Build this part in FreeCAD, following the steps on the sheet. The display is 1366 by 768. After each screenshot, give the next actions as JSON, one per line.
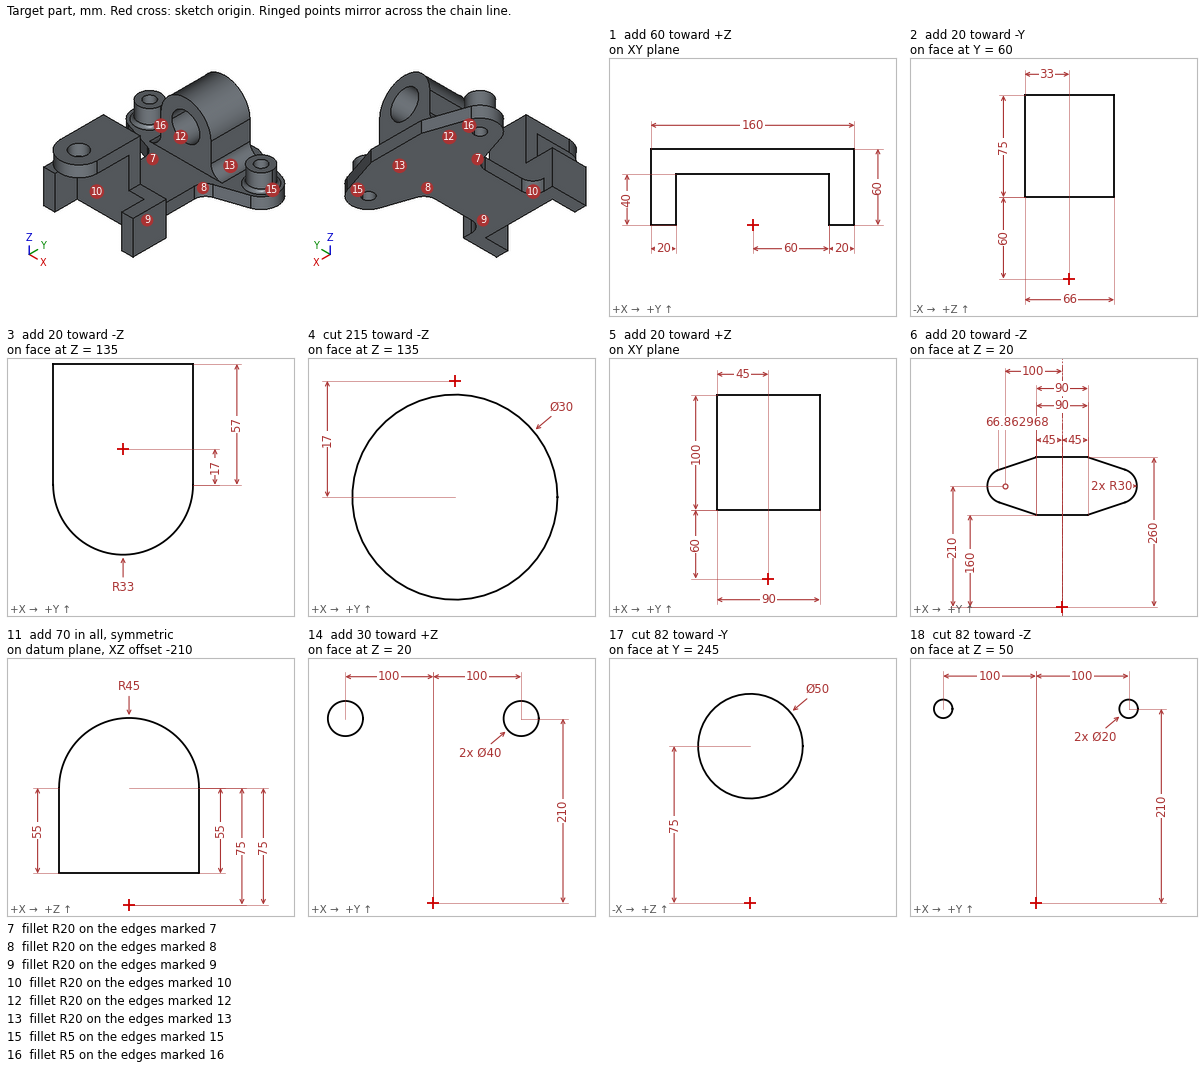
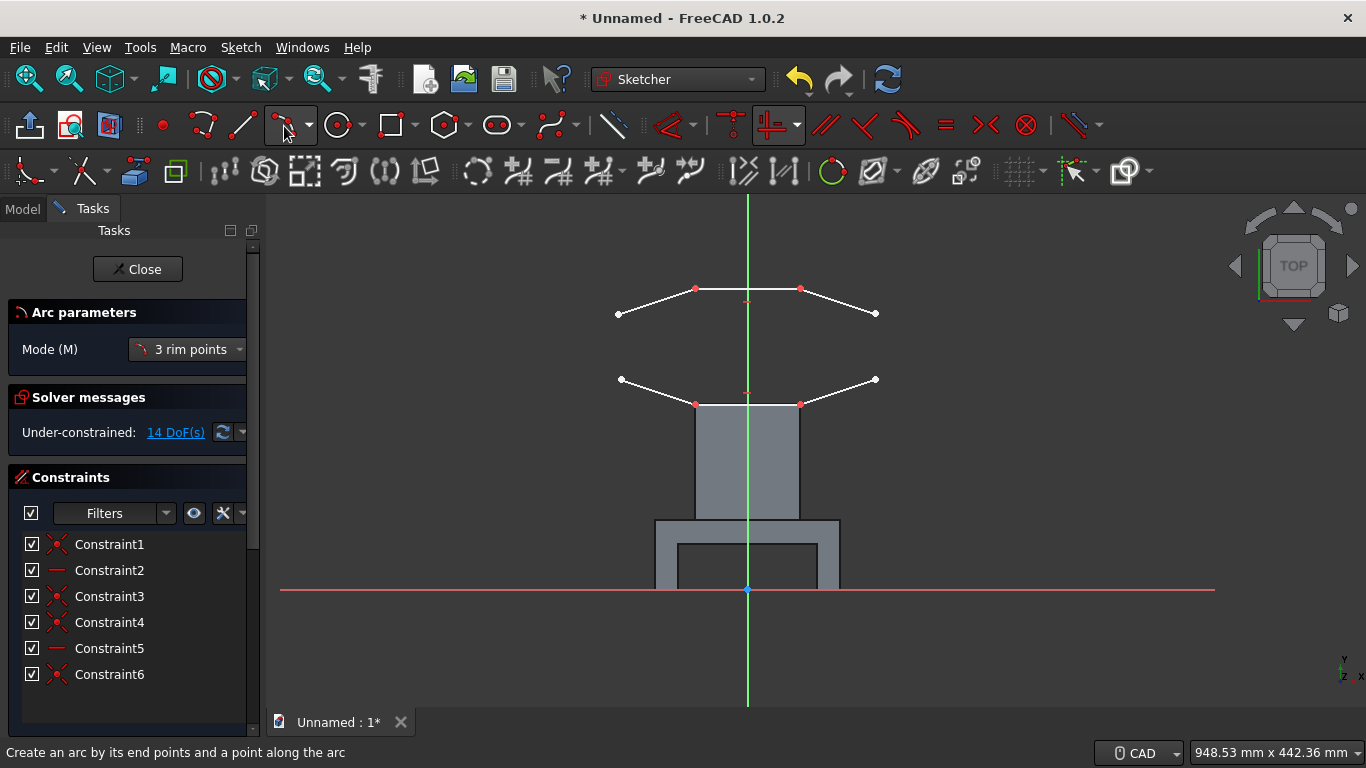
{"action": "left_click", "coordinate": [618, 315]}
{"action": "left_click", "coordinate": [621, 380]}
{"action": "left_click", "coordinate": [597, 348]}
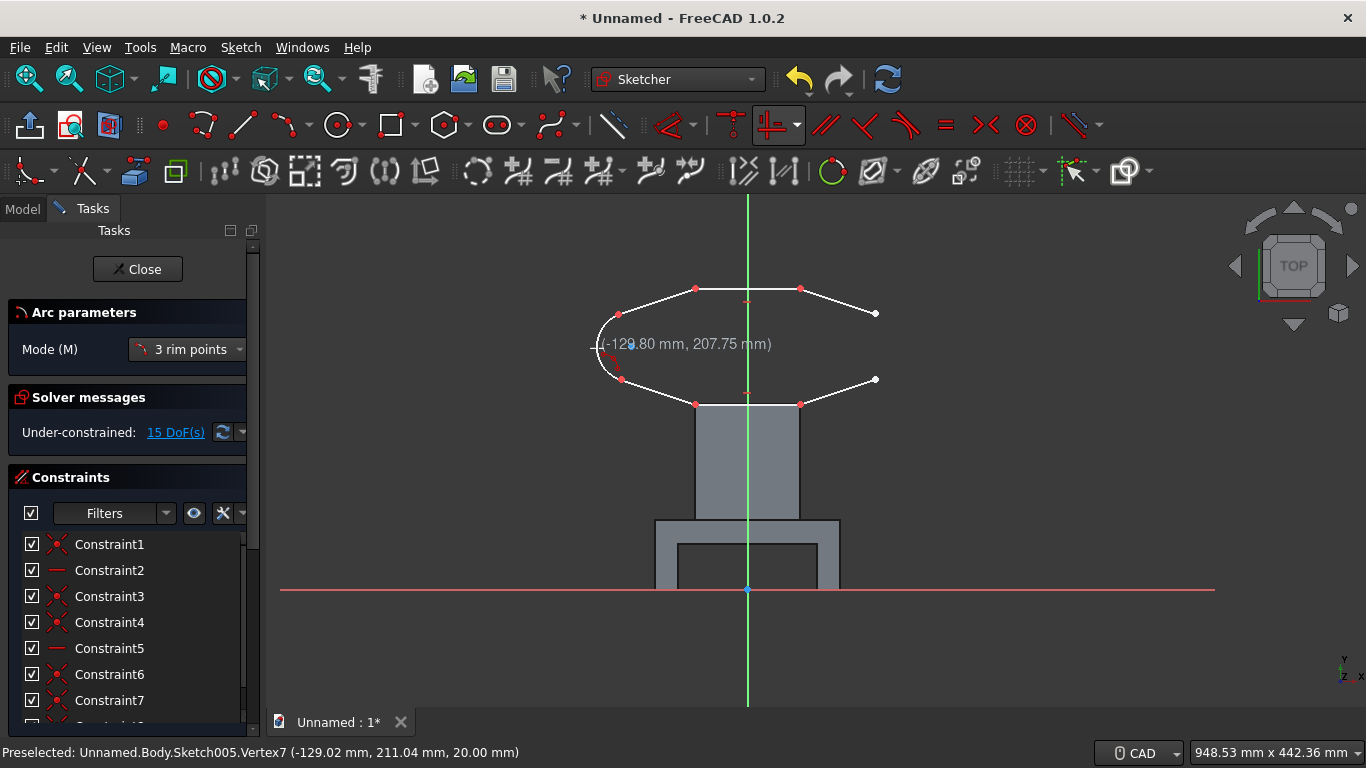
{"action": "left_click", "coordinate": [875, 380]}
{"action": "left_click", "coordinate": [875, 314]}
{"action": "left_click", "coordinate": [898, 346]}
{"action": "key", "text": "Escape"}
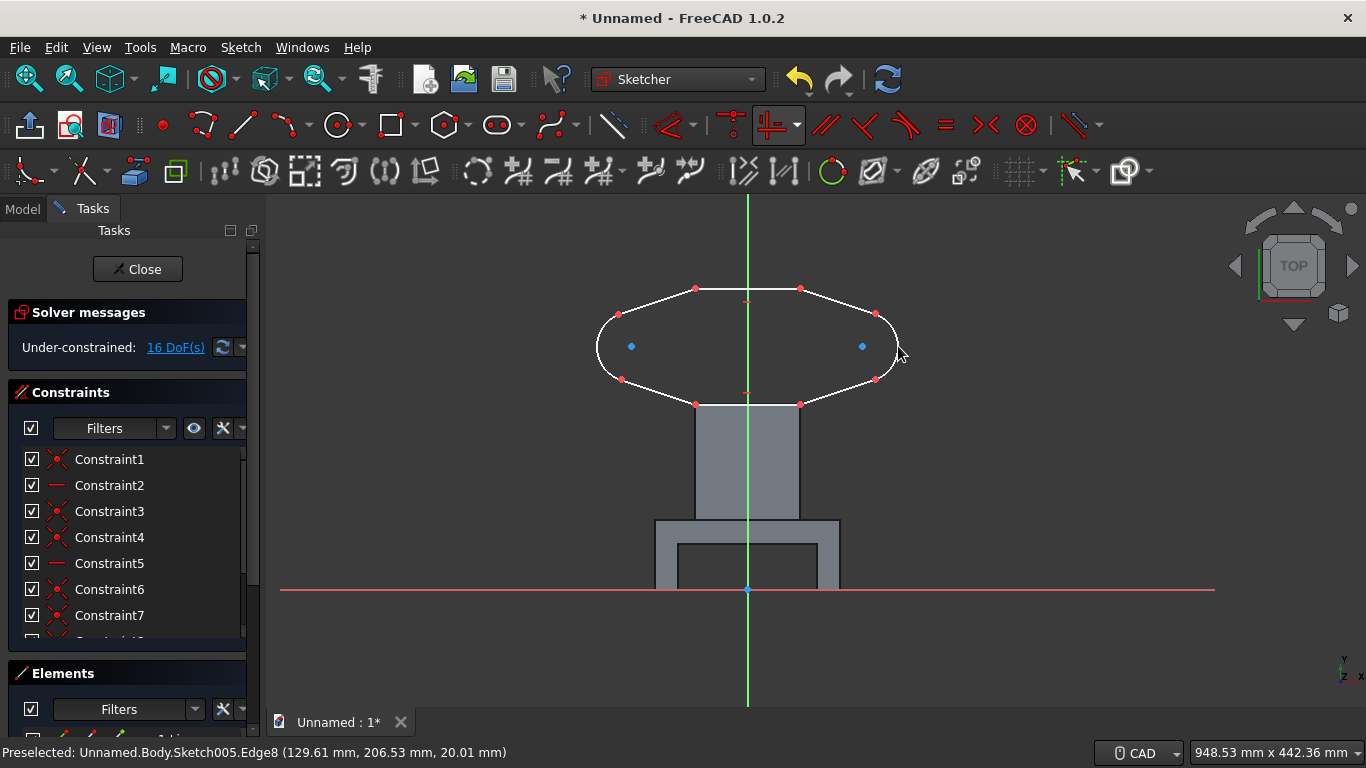
{"action": "left_click", "coordinate": [853, 306]}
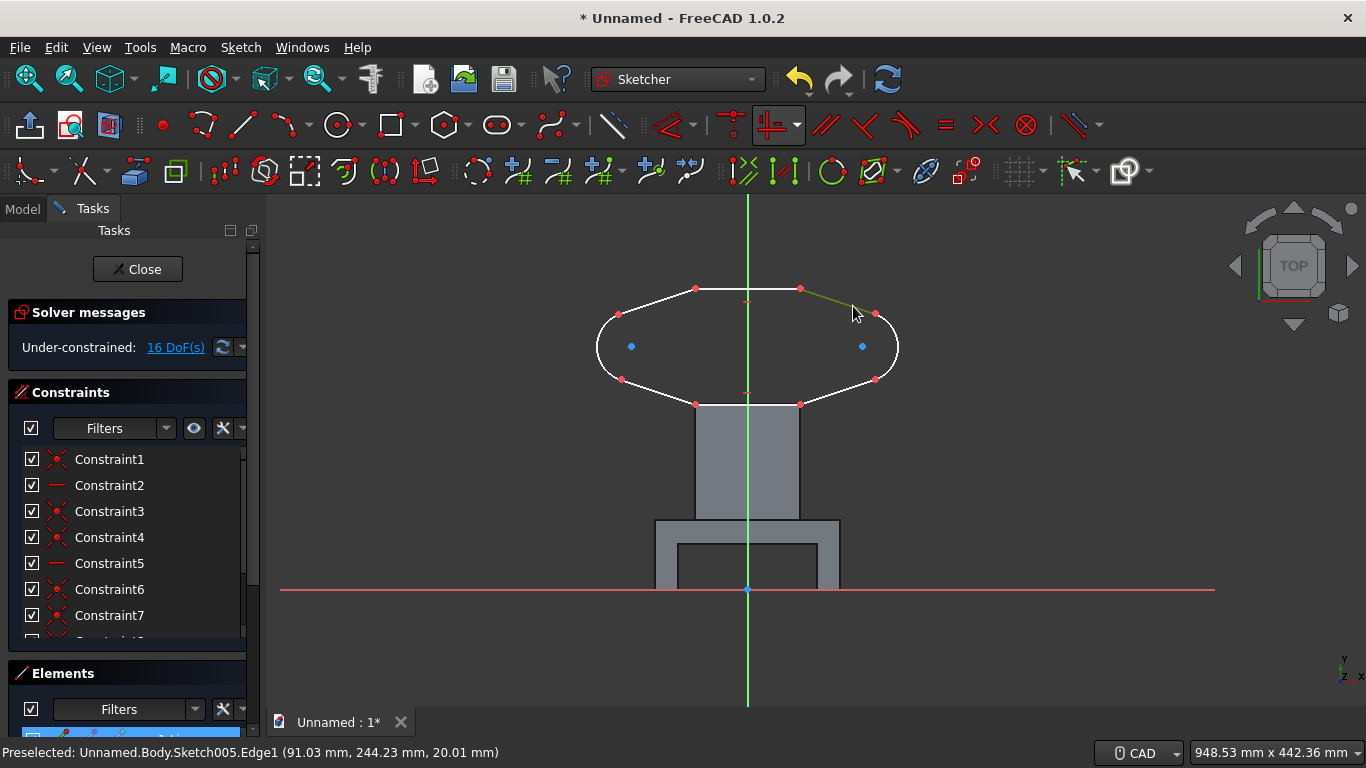
{"action": "left_click", "coordinate": [894, 363]}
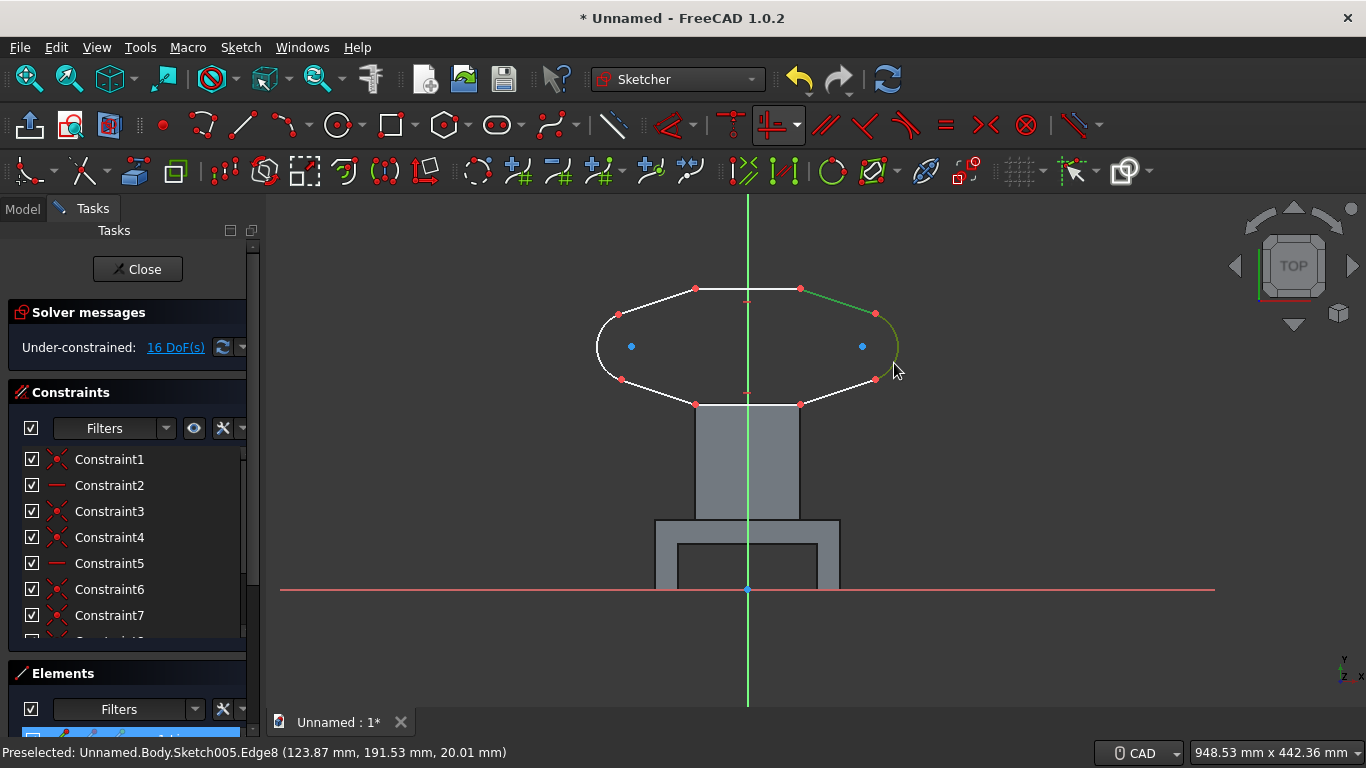
{"action": "key", "text": "t"}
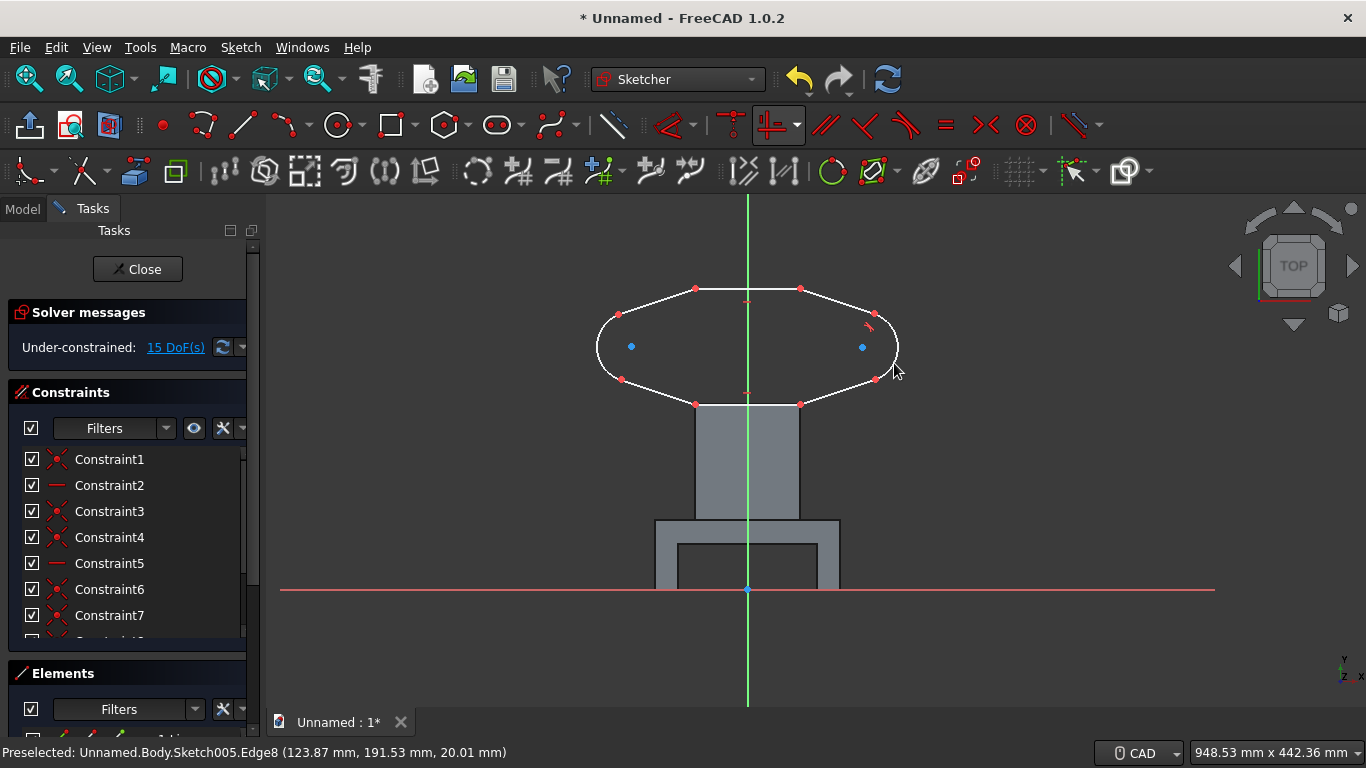
{"action": "left_click", "coordinate": [643, 387]}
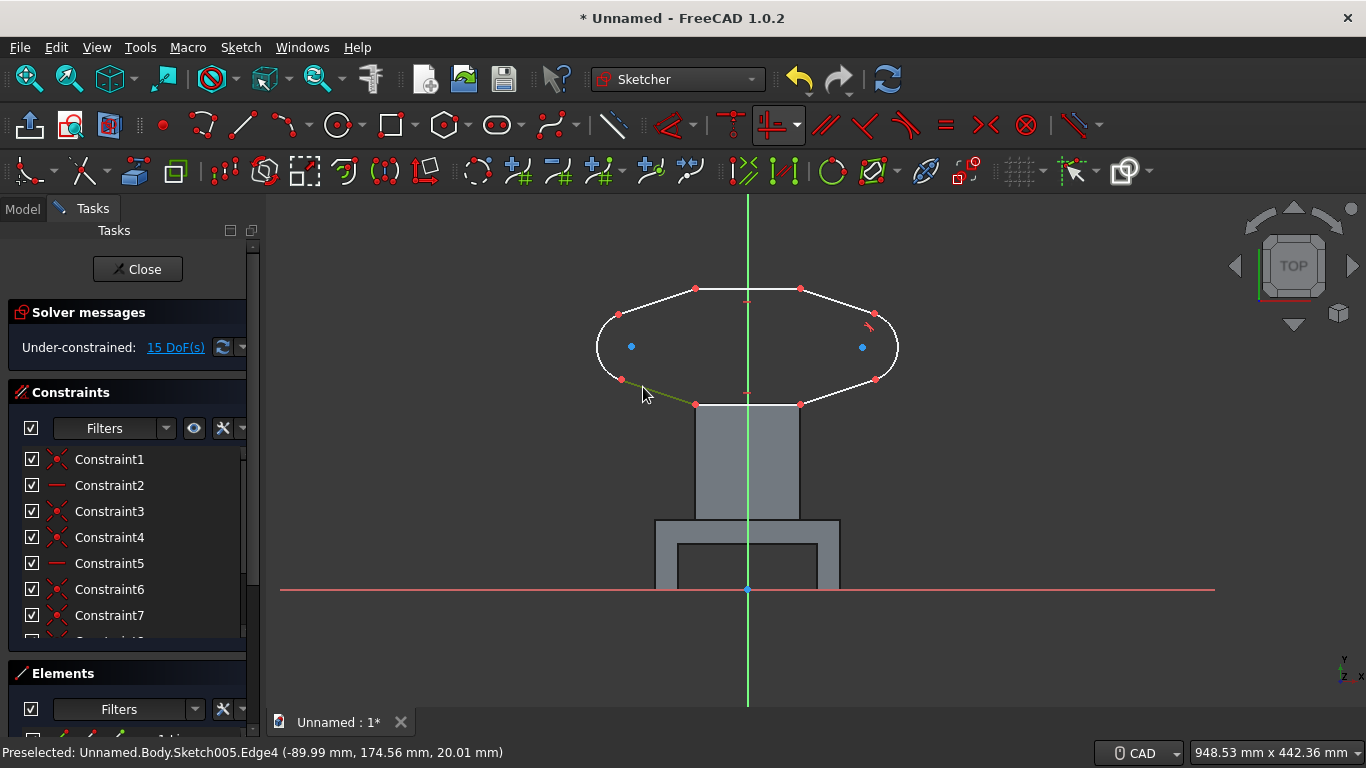
{"action": "left_click", "coordinate": [600, 332]}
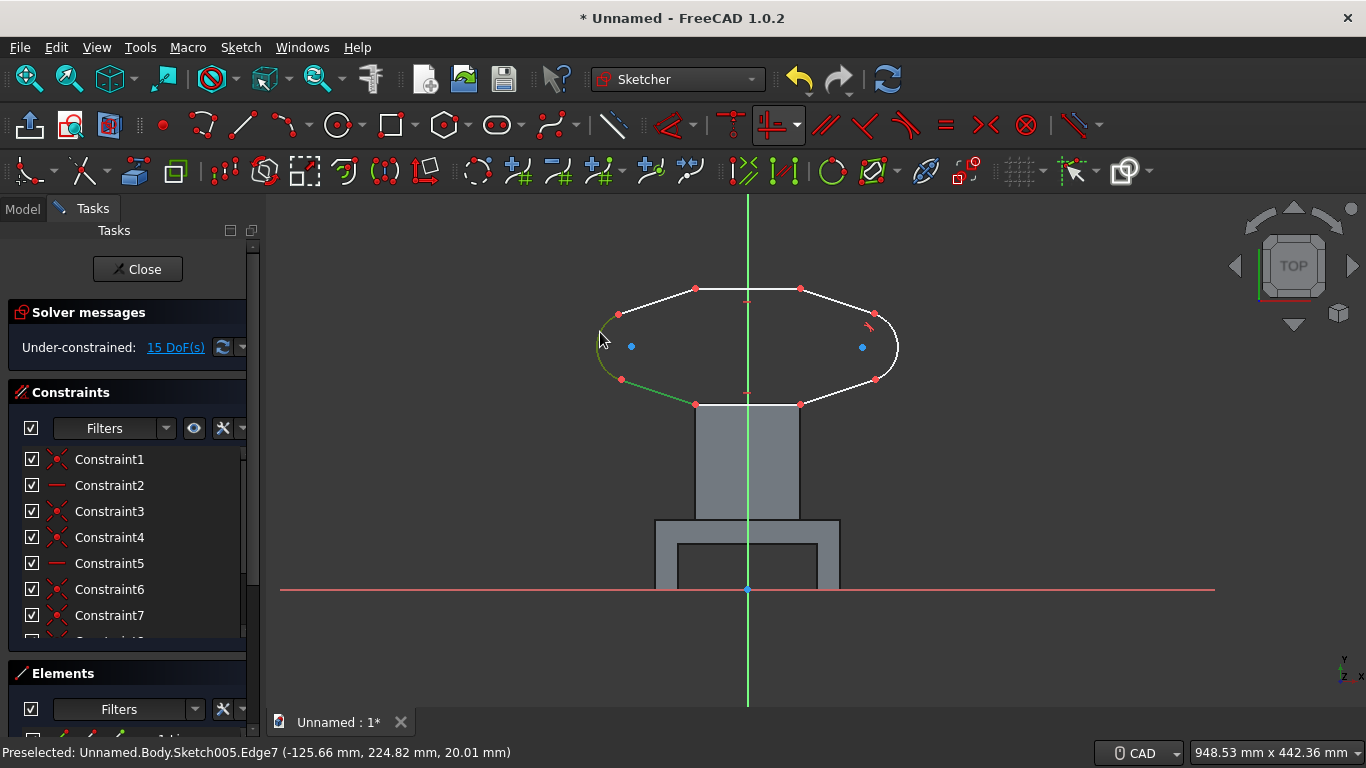
{"action": "key", "text": "t"}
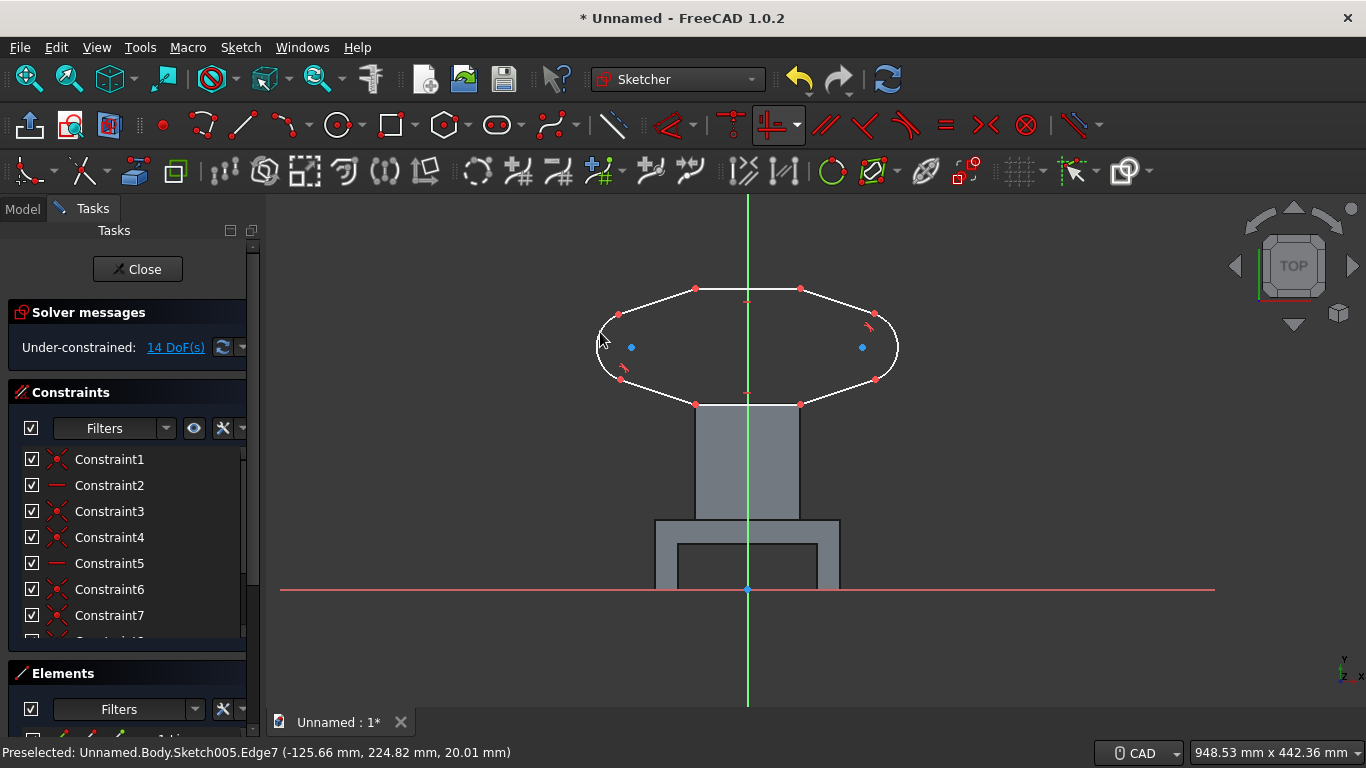
{"action": "left_click", "coordinate": [823, 397]}